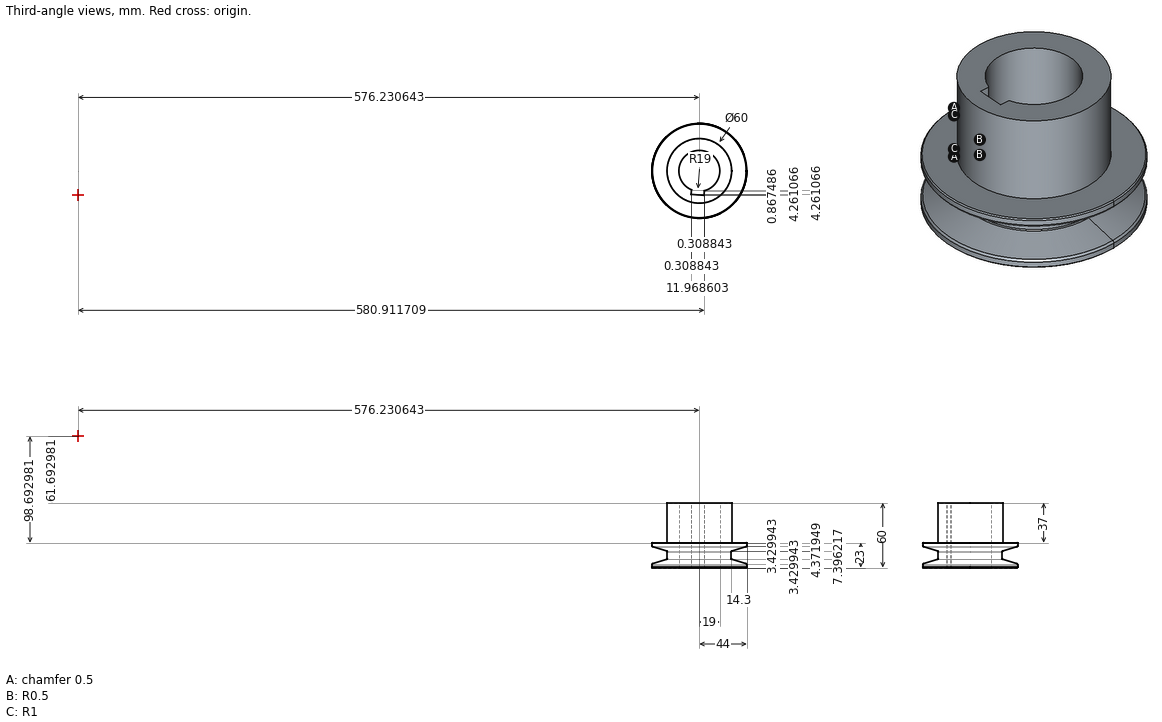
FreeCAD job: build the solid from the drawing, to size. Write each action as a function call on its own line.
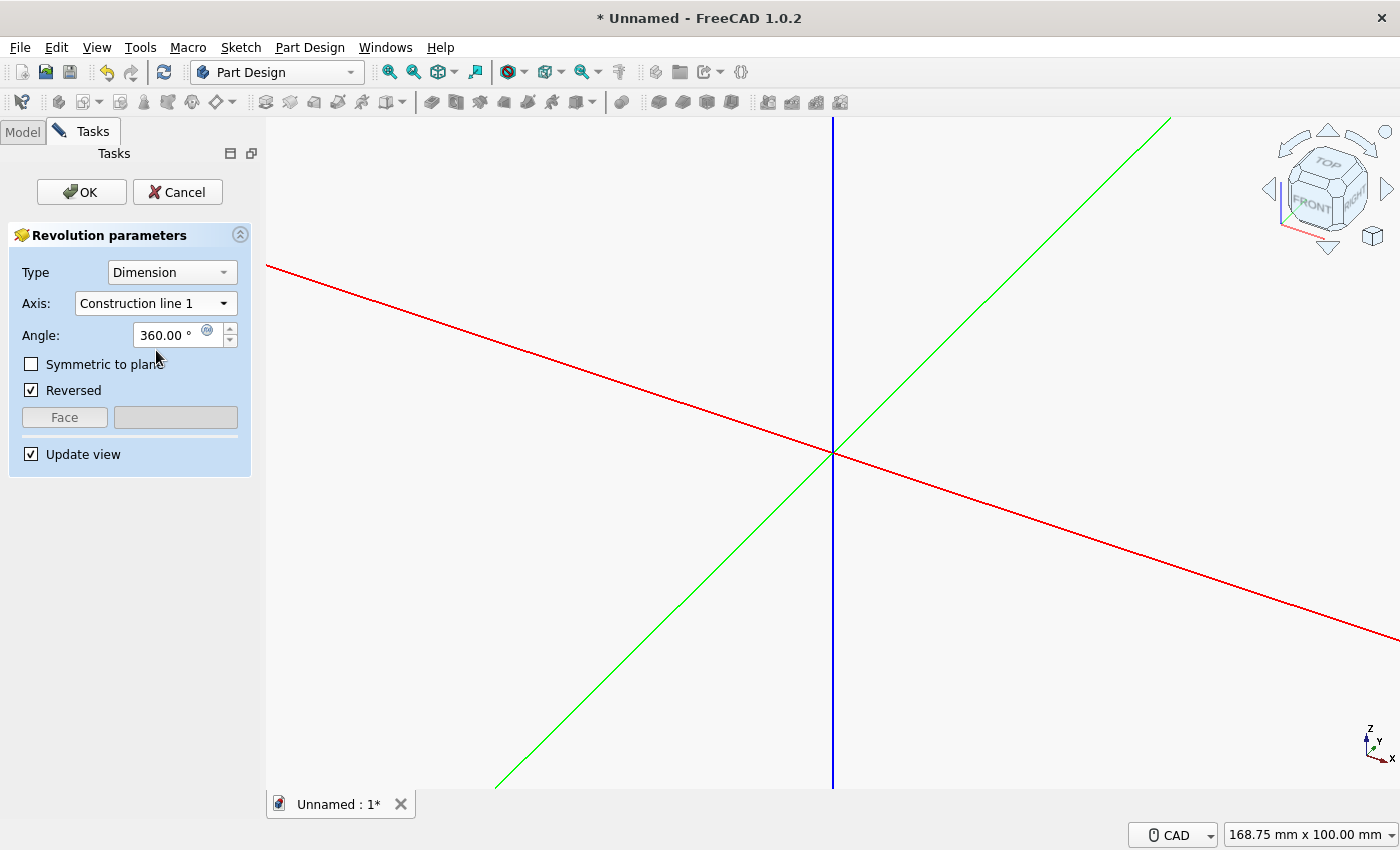
click(82, 192)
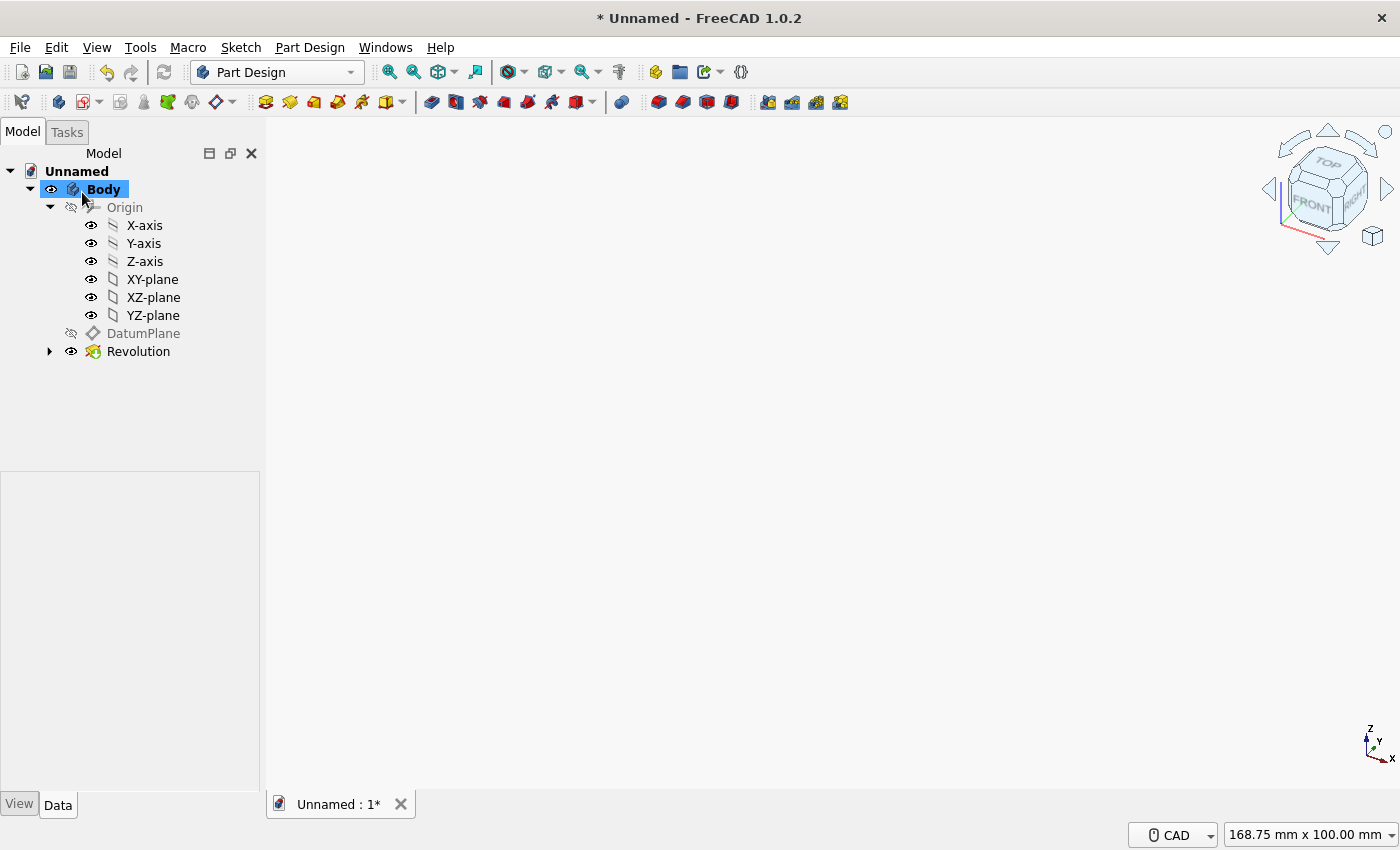
click(390, 72)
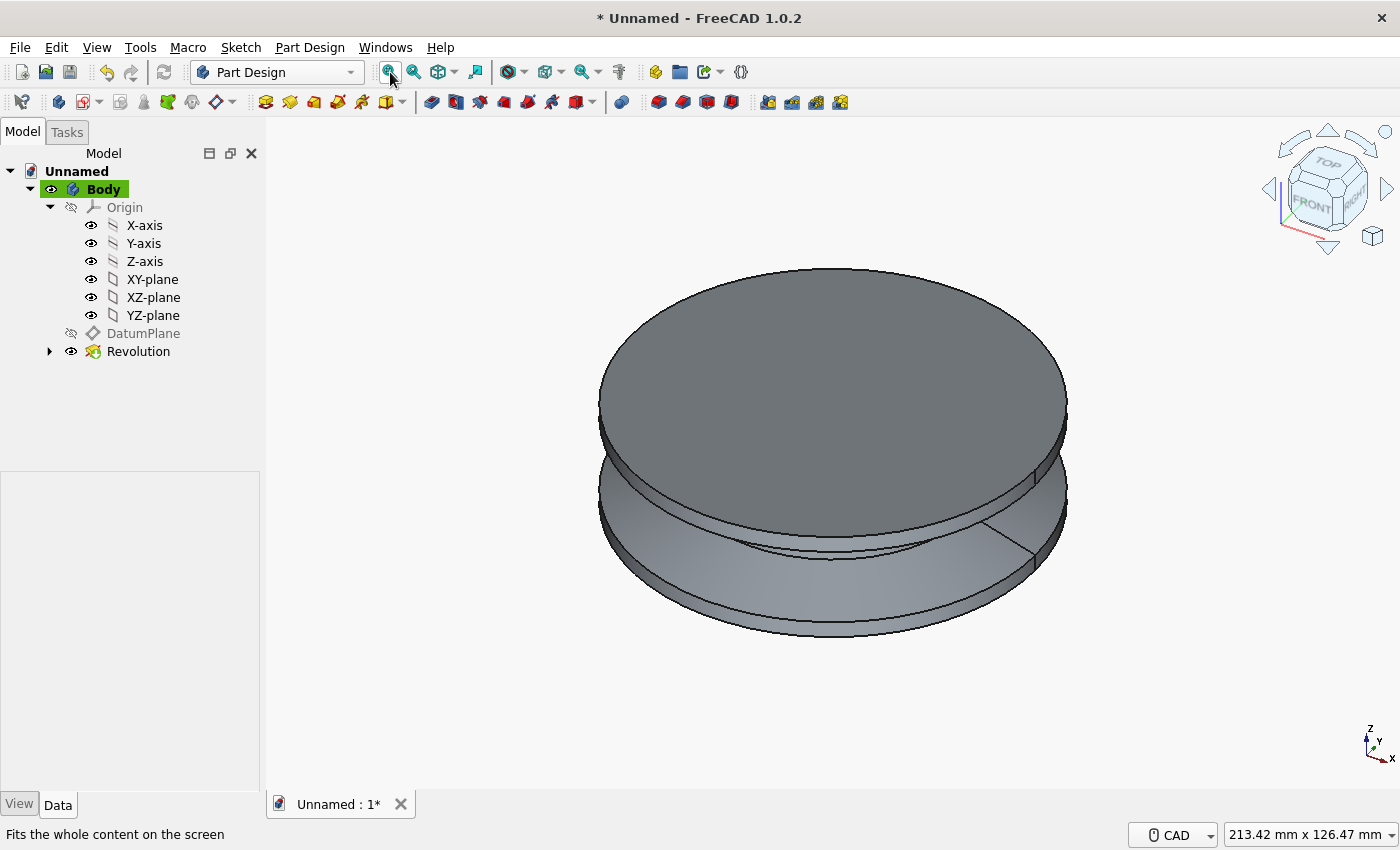
click(833, 402)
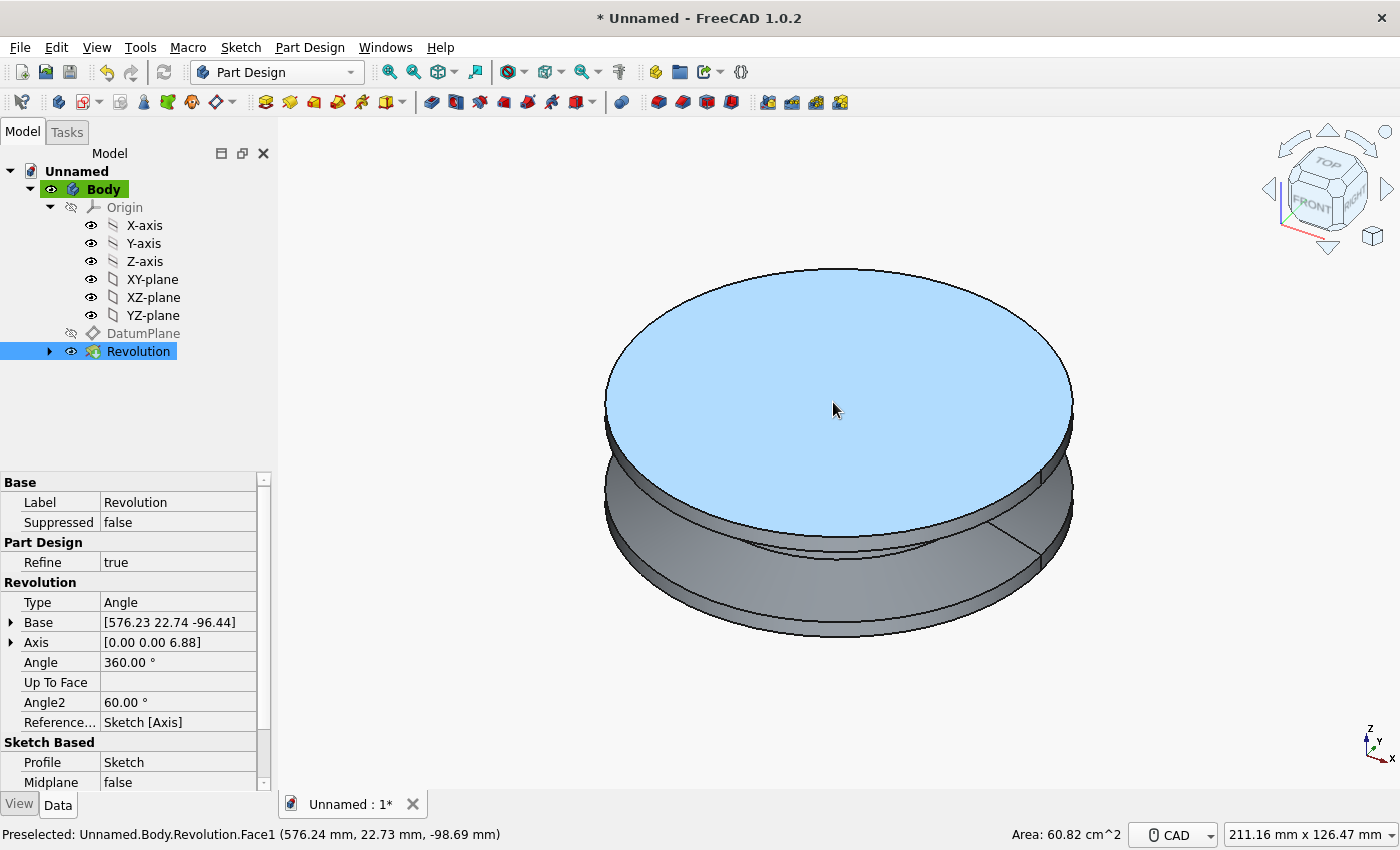
click(84, 102)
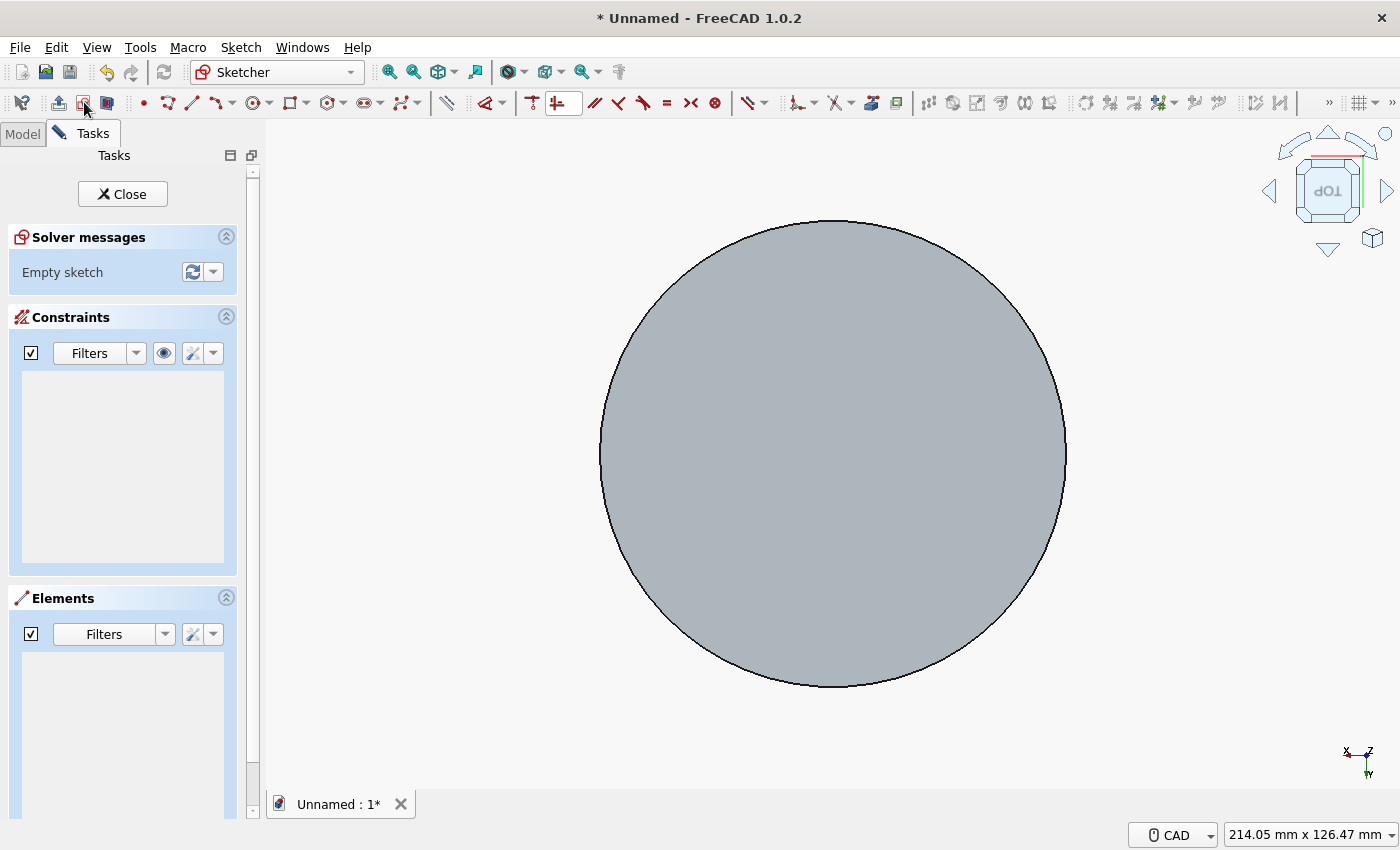
scroll(972, 454, up, 2)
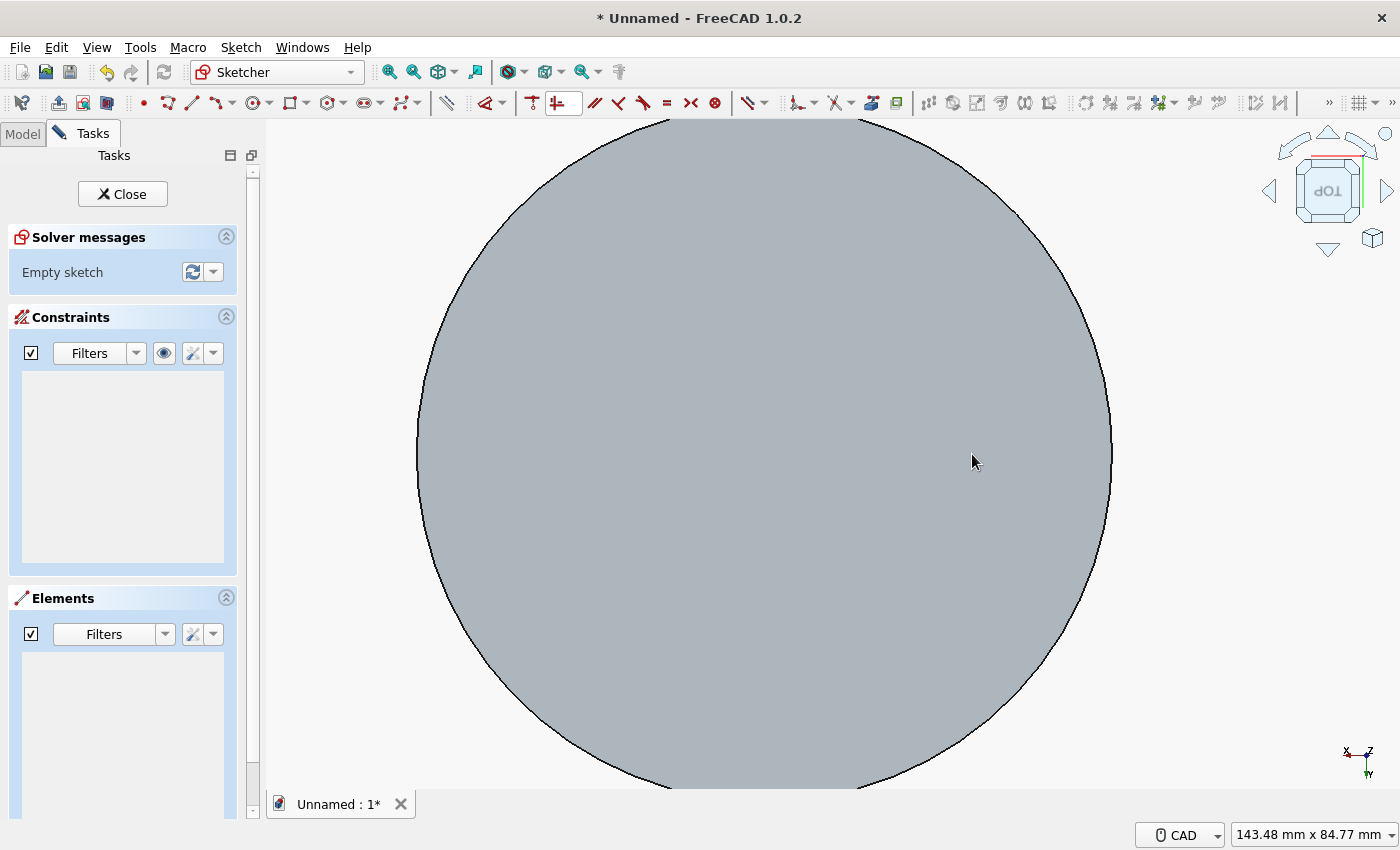
click(254, 104)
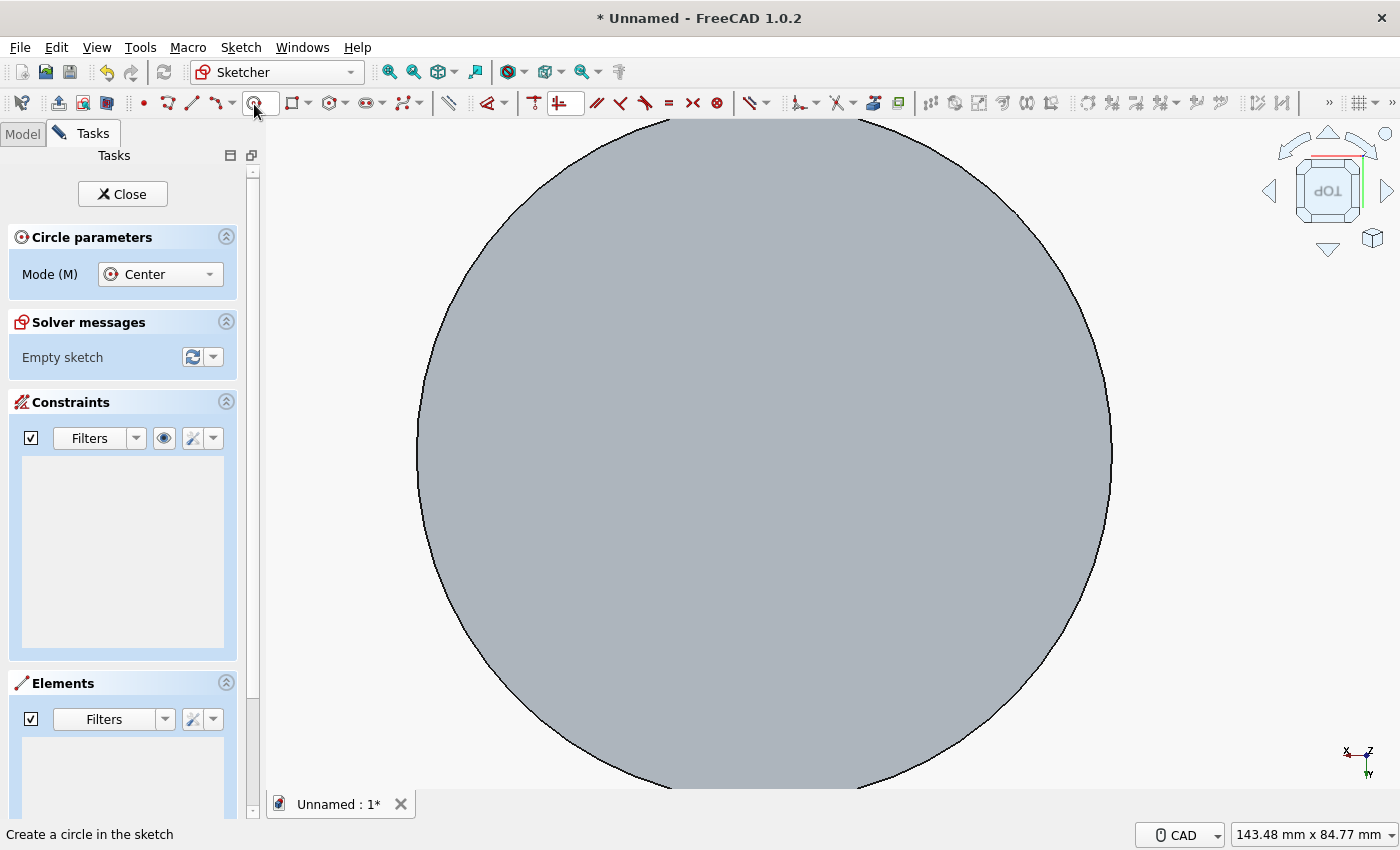
click(764, 454)
click(932, 286)
key(Escape)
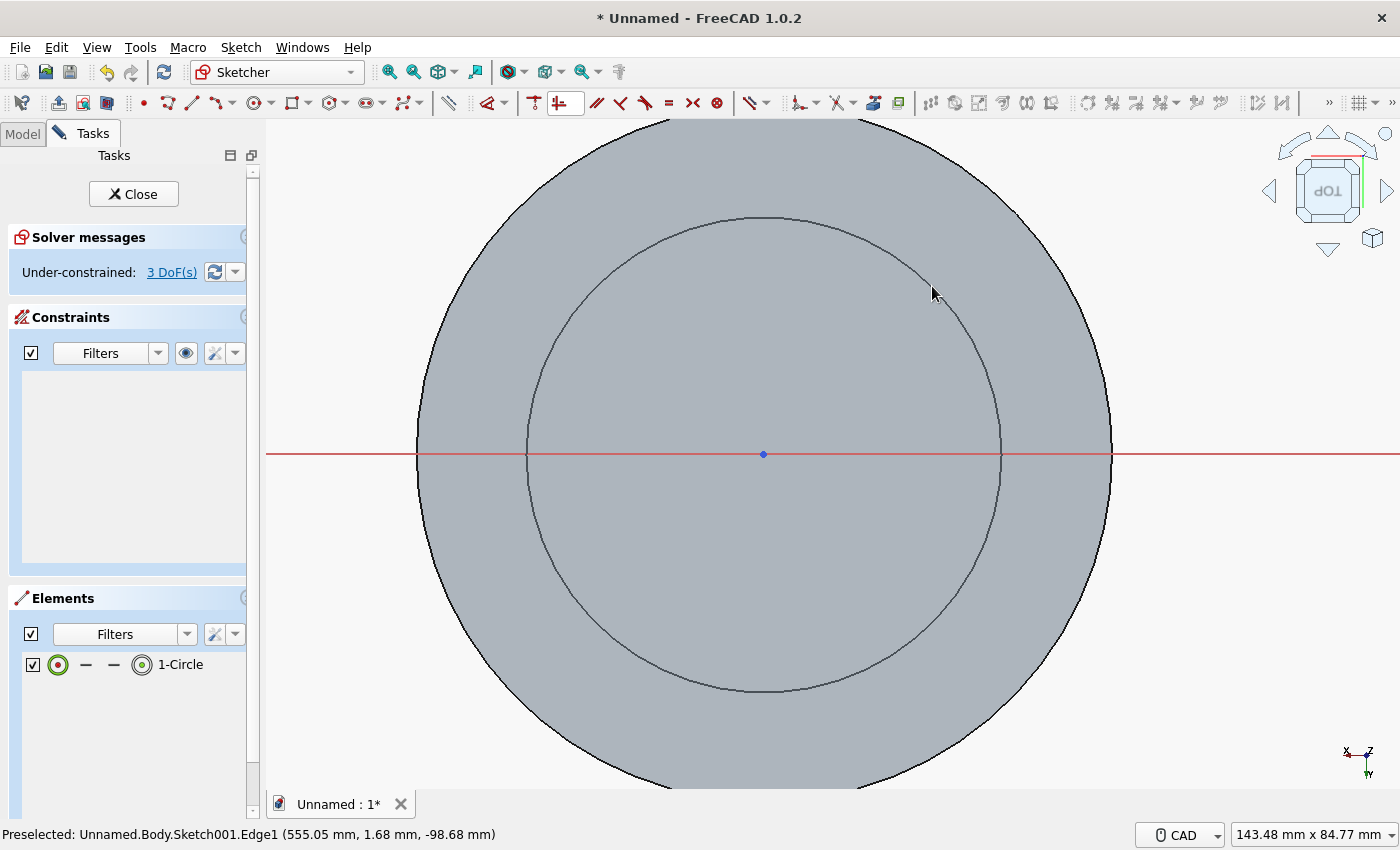
click(764, 455)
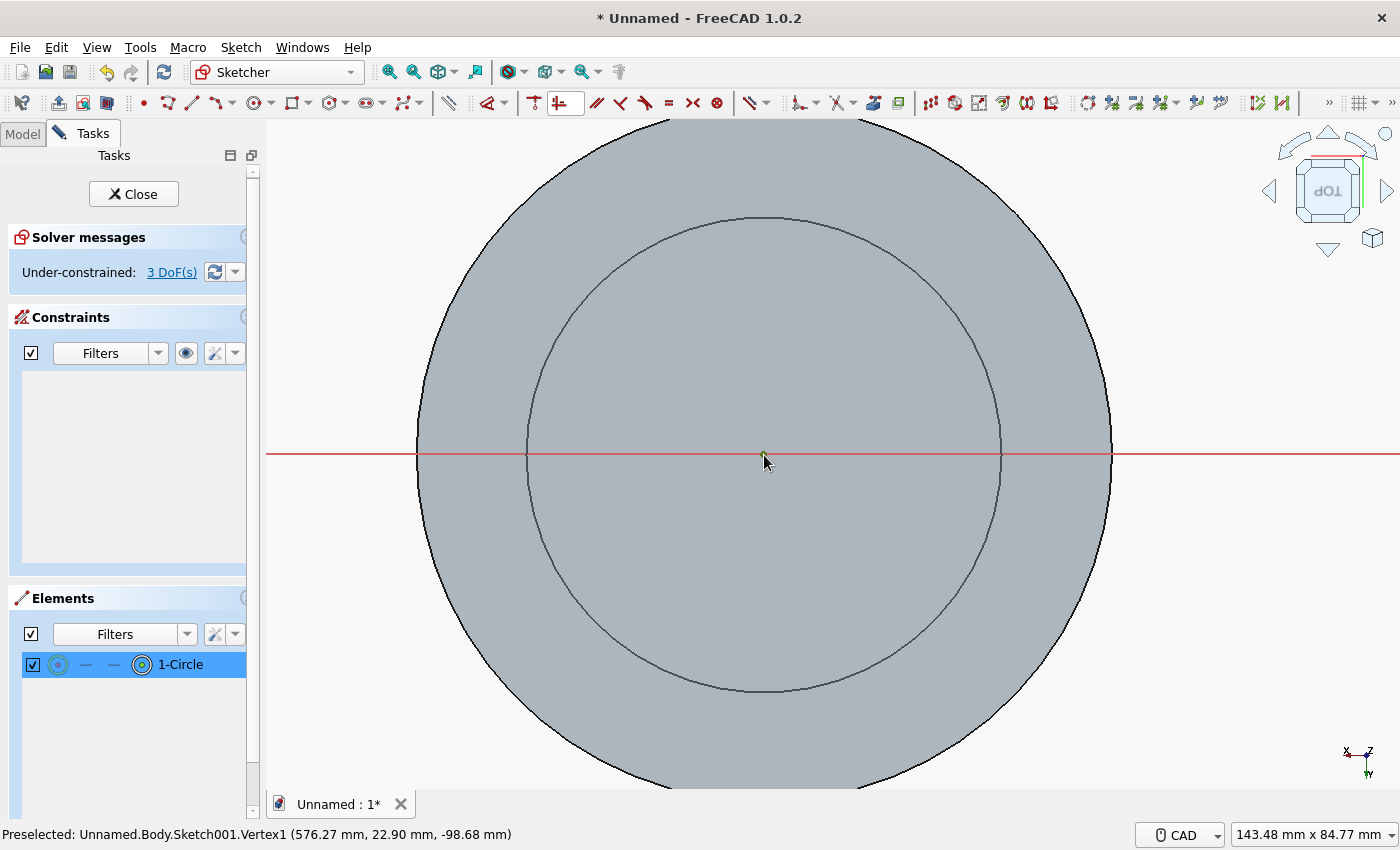
click(361, 454)